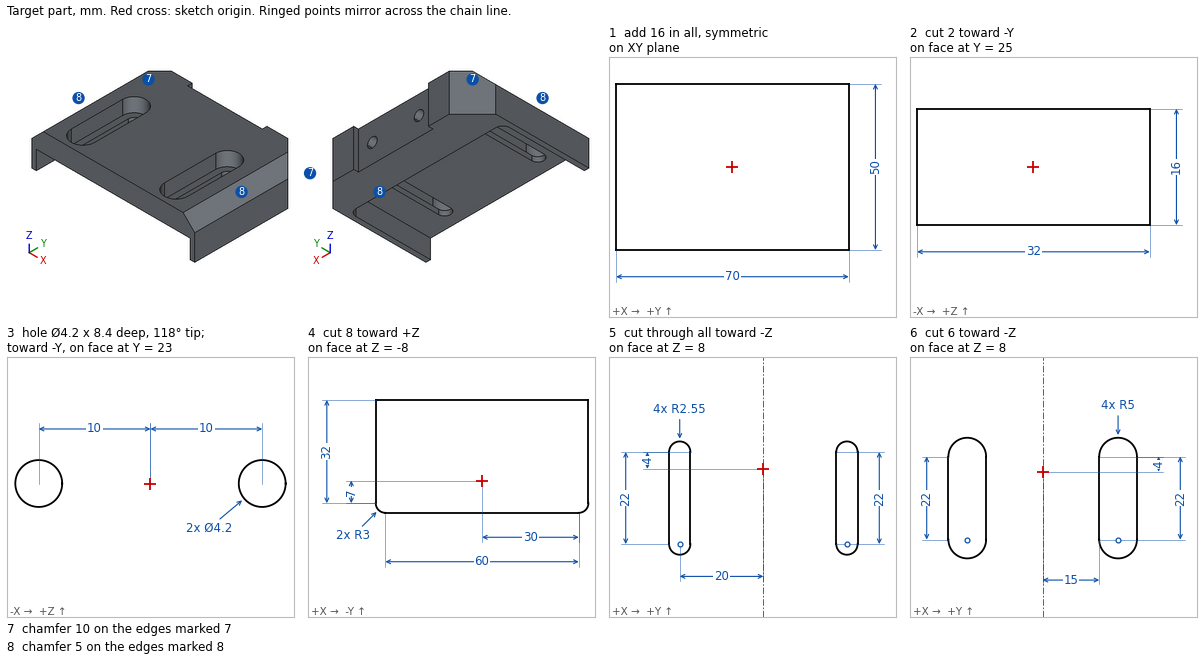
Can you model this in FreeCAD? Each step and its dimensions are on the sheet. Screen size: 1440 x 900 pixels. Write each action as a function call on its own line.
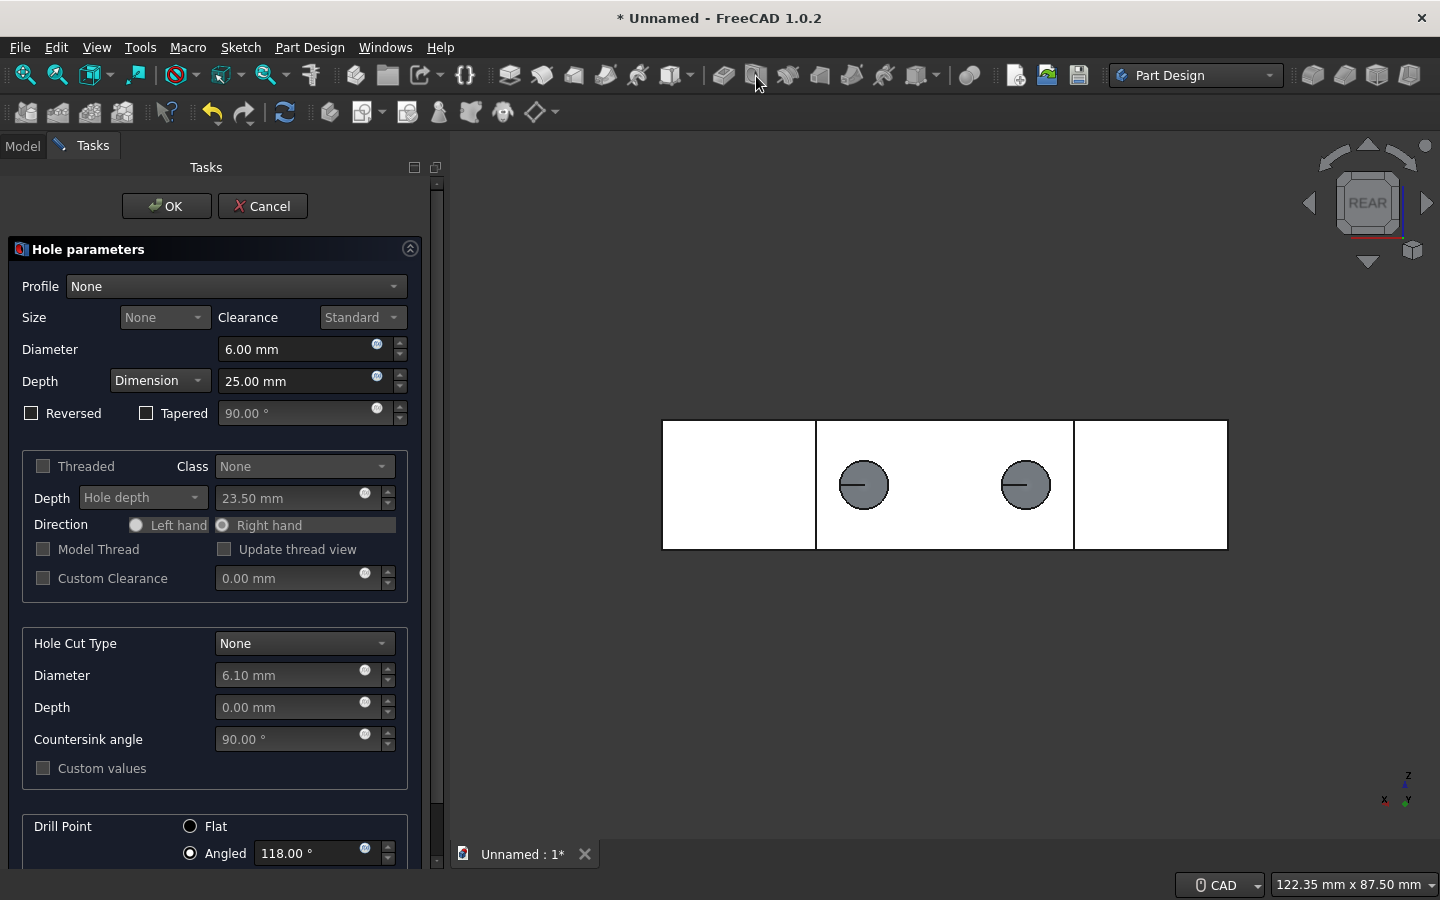
triple_click(305, 349)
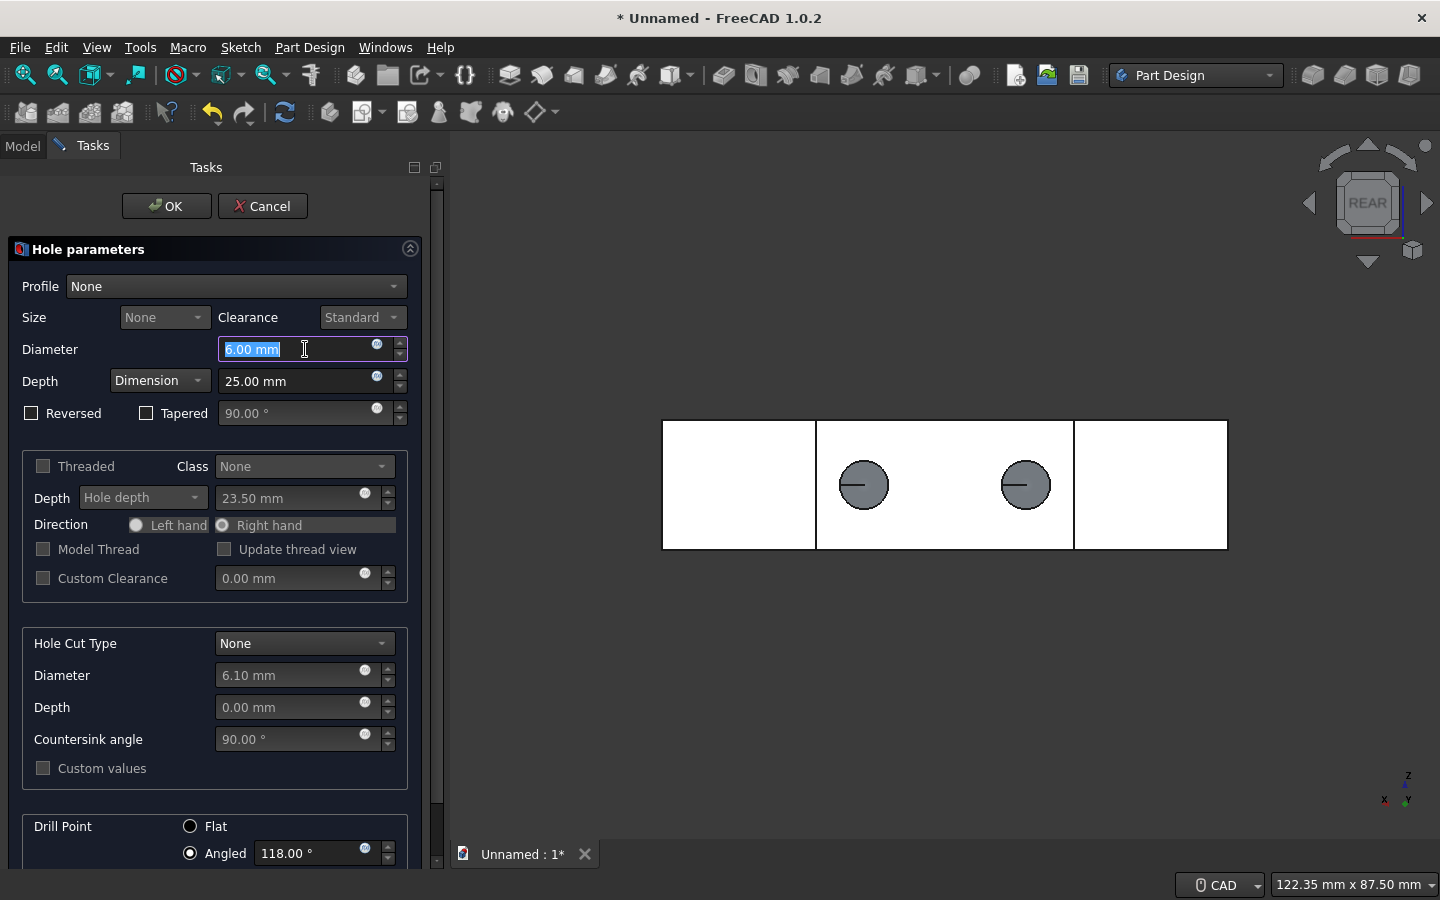
text(4.2)
key(Tab)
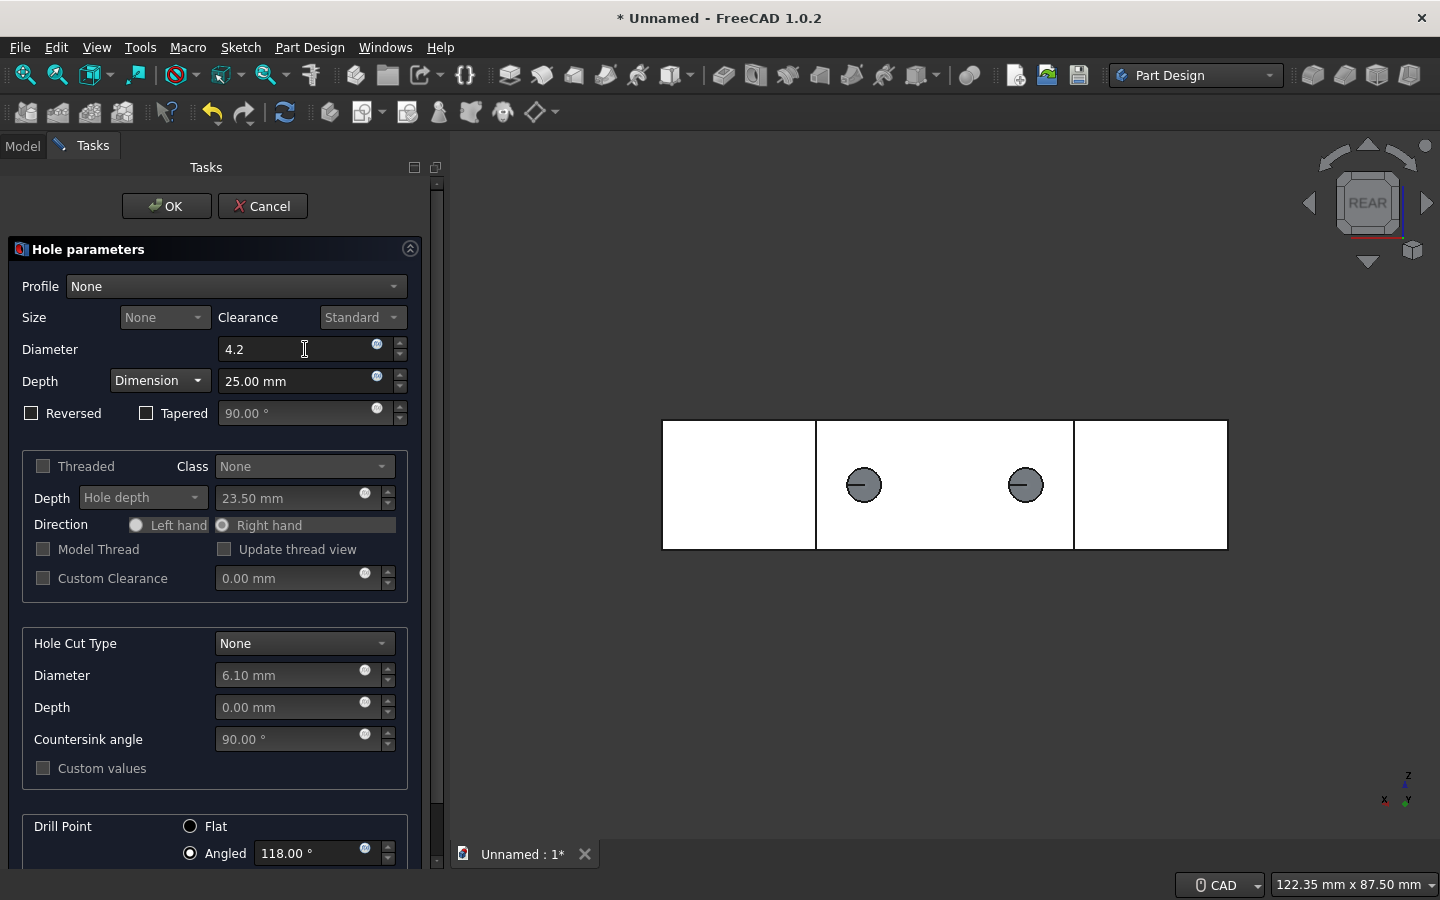
triple_click(305, 381)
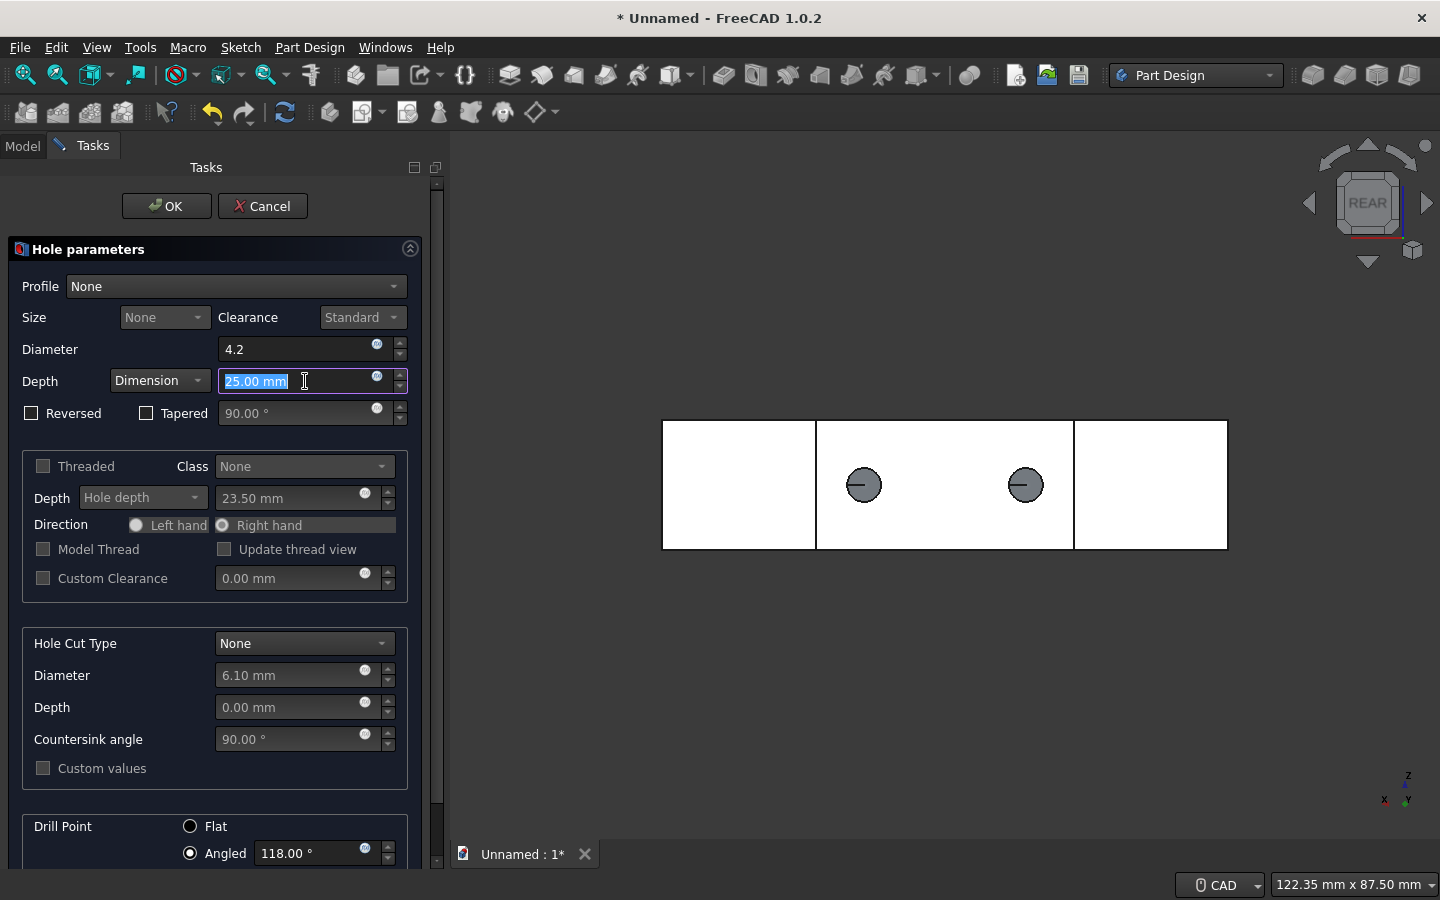
text(8.4)
key(Tab)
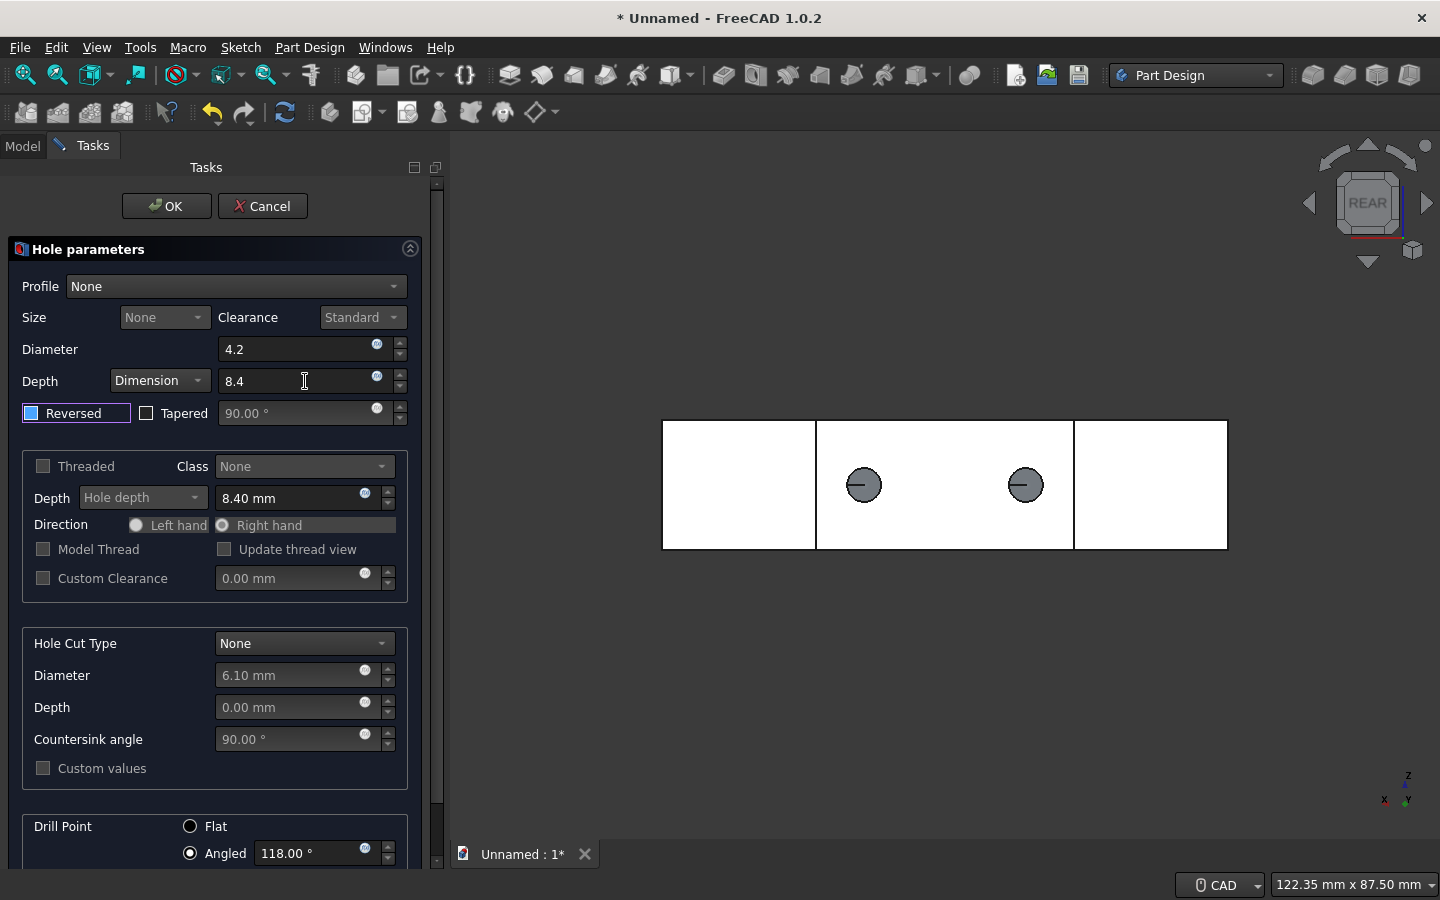
click(167, 206)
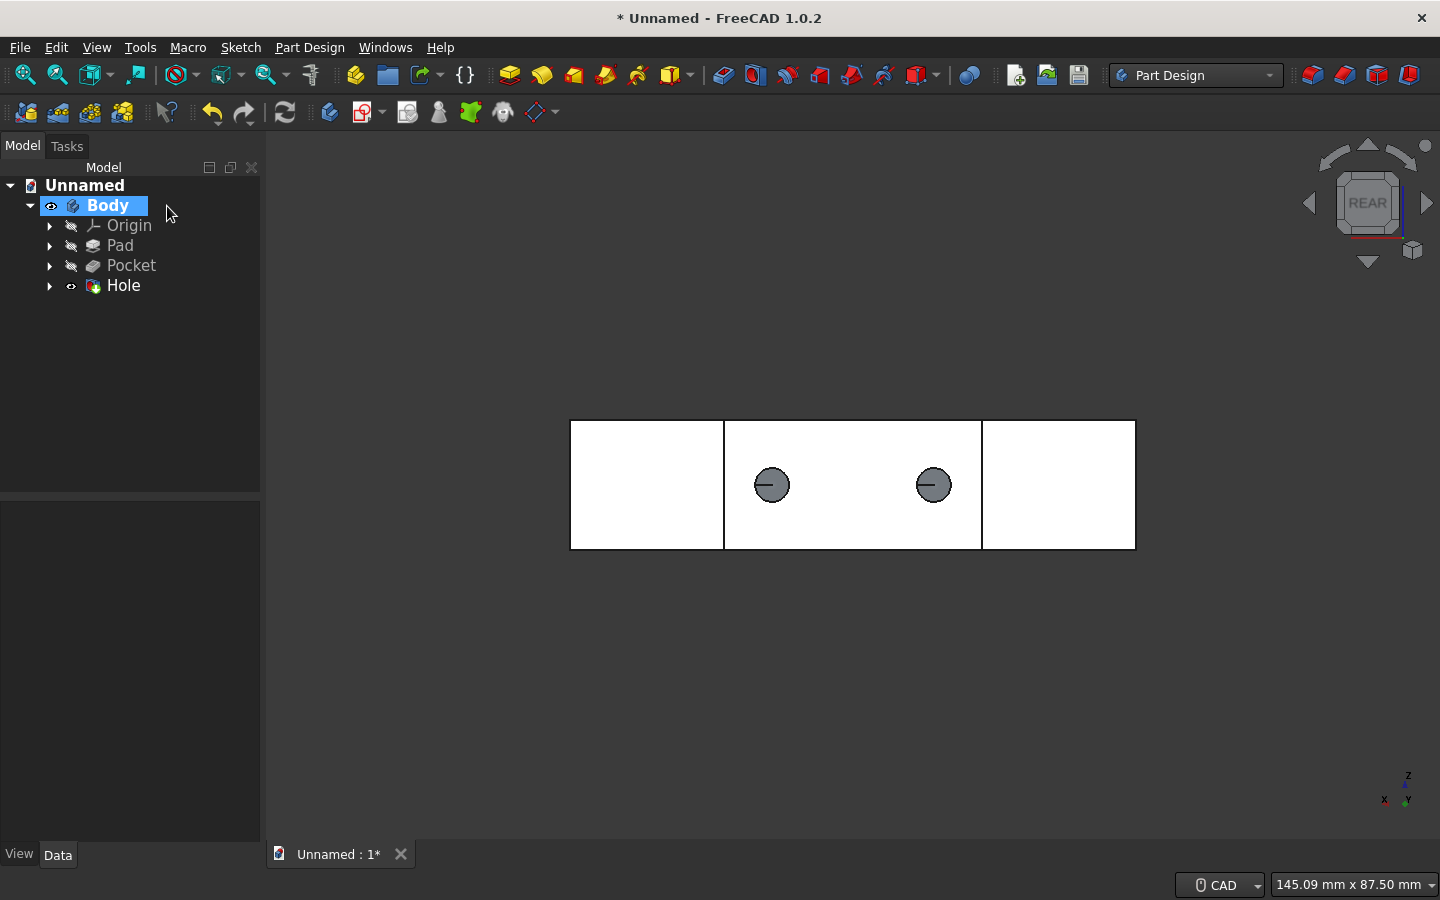
key(5)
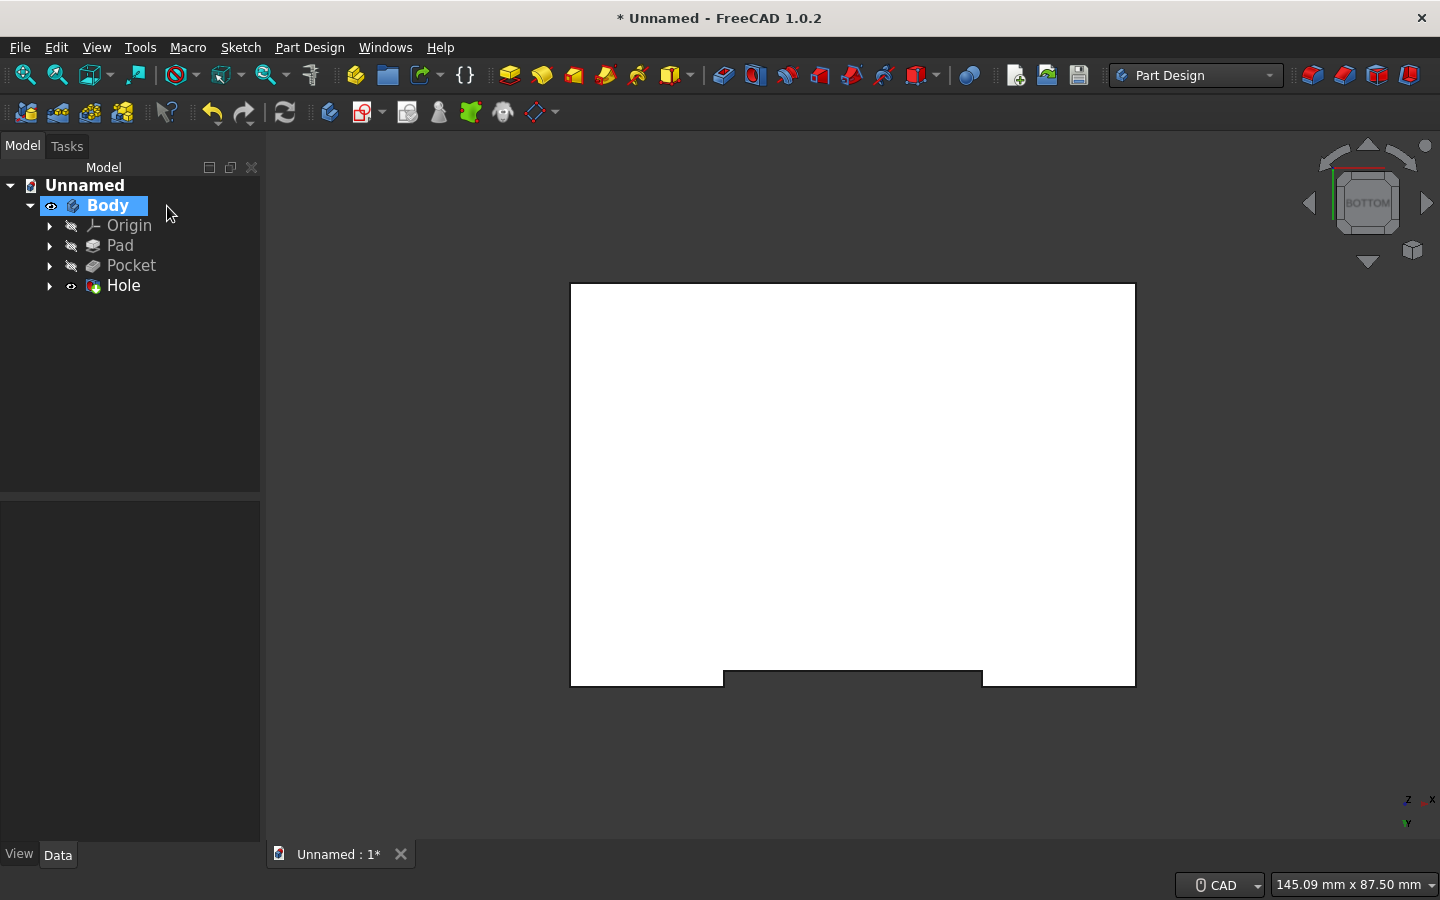
click(934, 484)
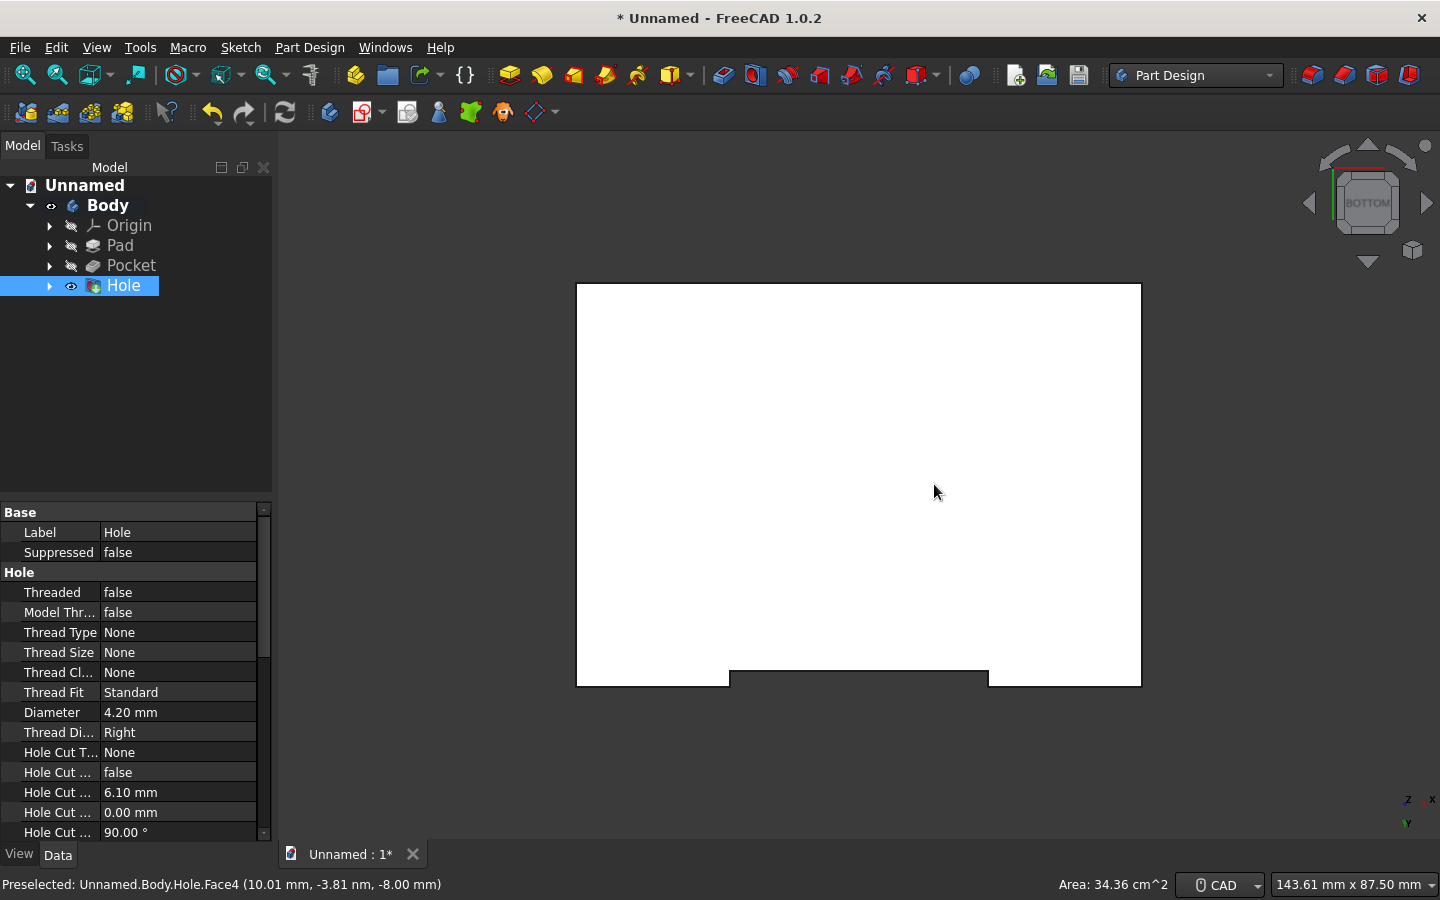
click(362, 112)